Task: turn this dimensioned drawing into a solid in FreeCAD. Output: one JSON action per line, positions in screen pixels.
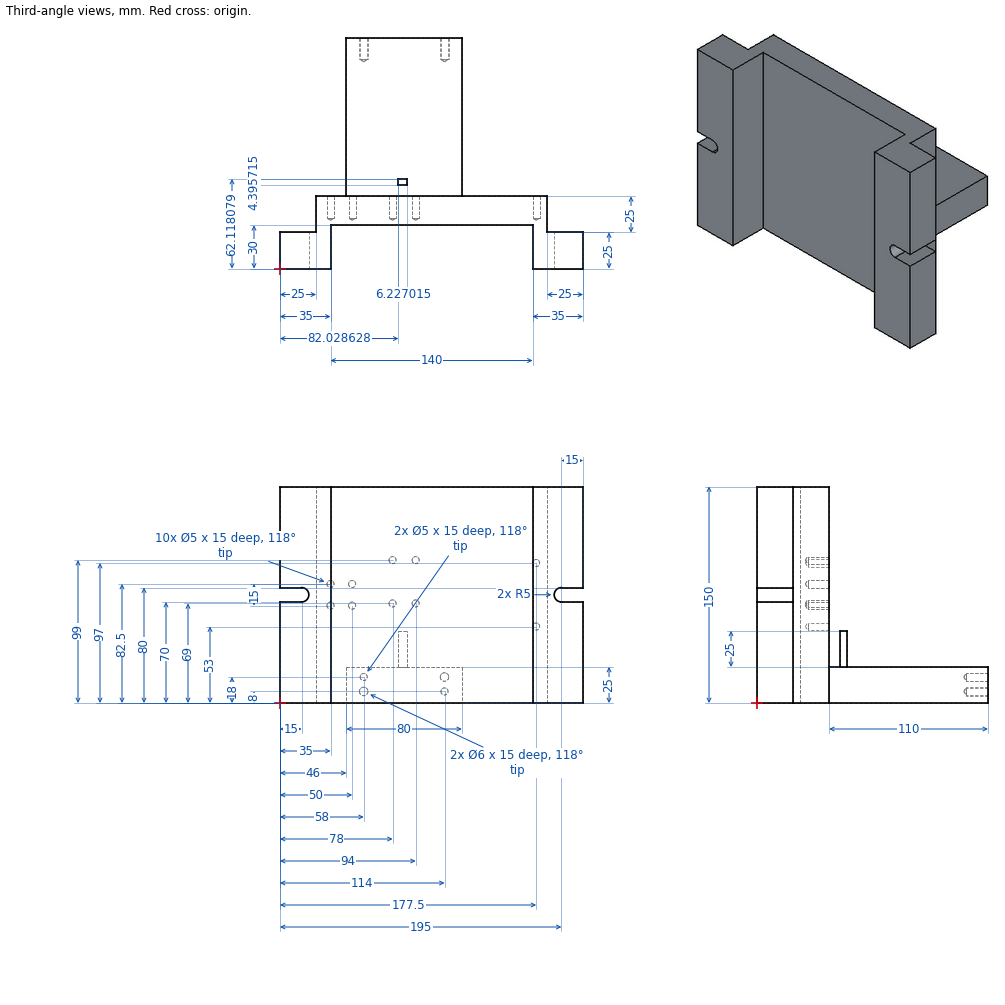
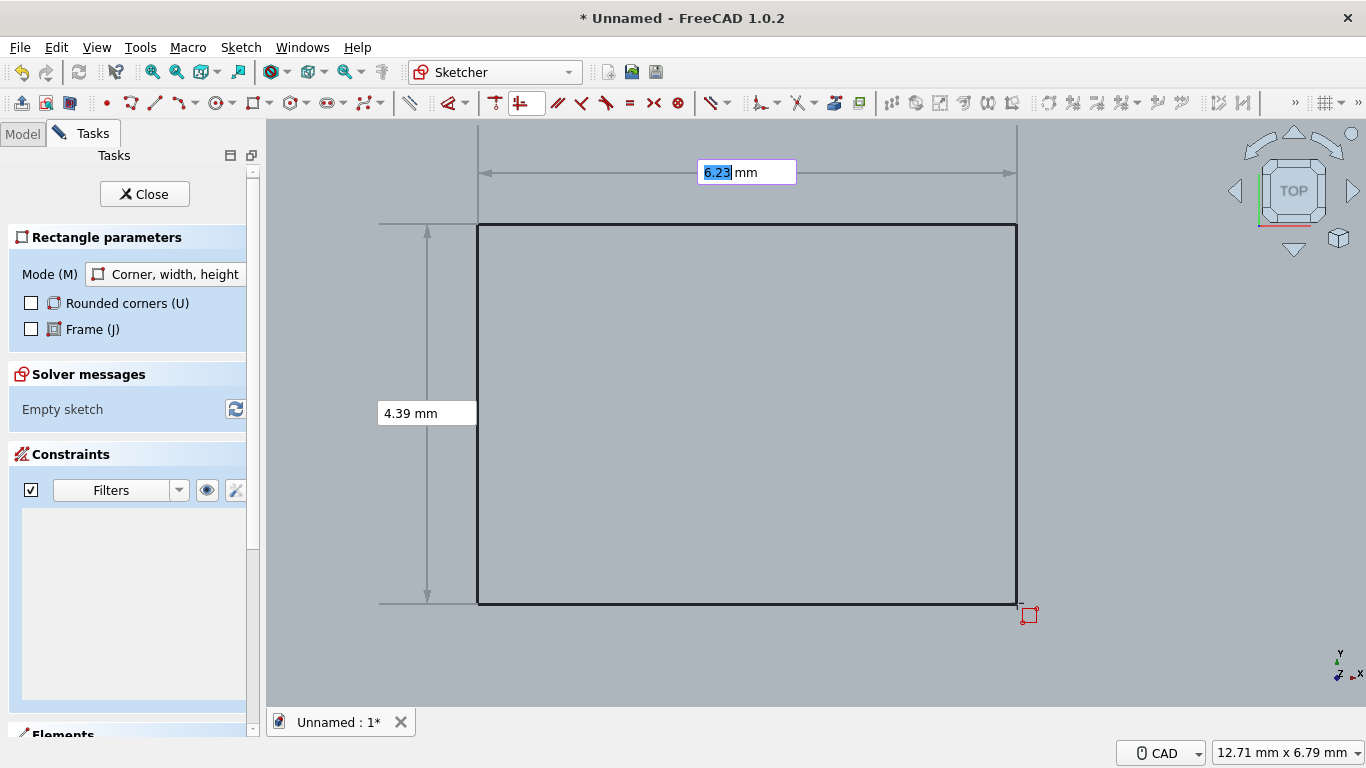
{"action": "type", "text": "6.227015"}
{"action": "key", "text": "Tab"}
{"action": "type", "text": "4.395715"}
{"action": "key", "text": "Return"}
{"action": "key", "text": "Escape"}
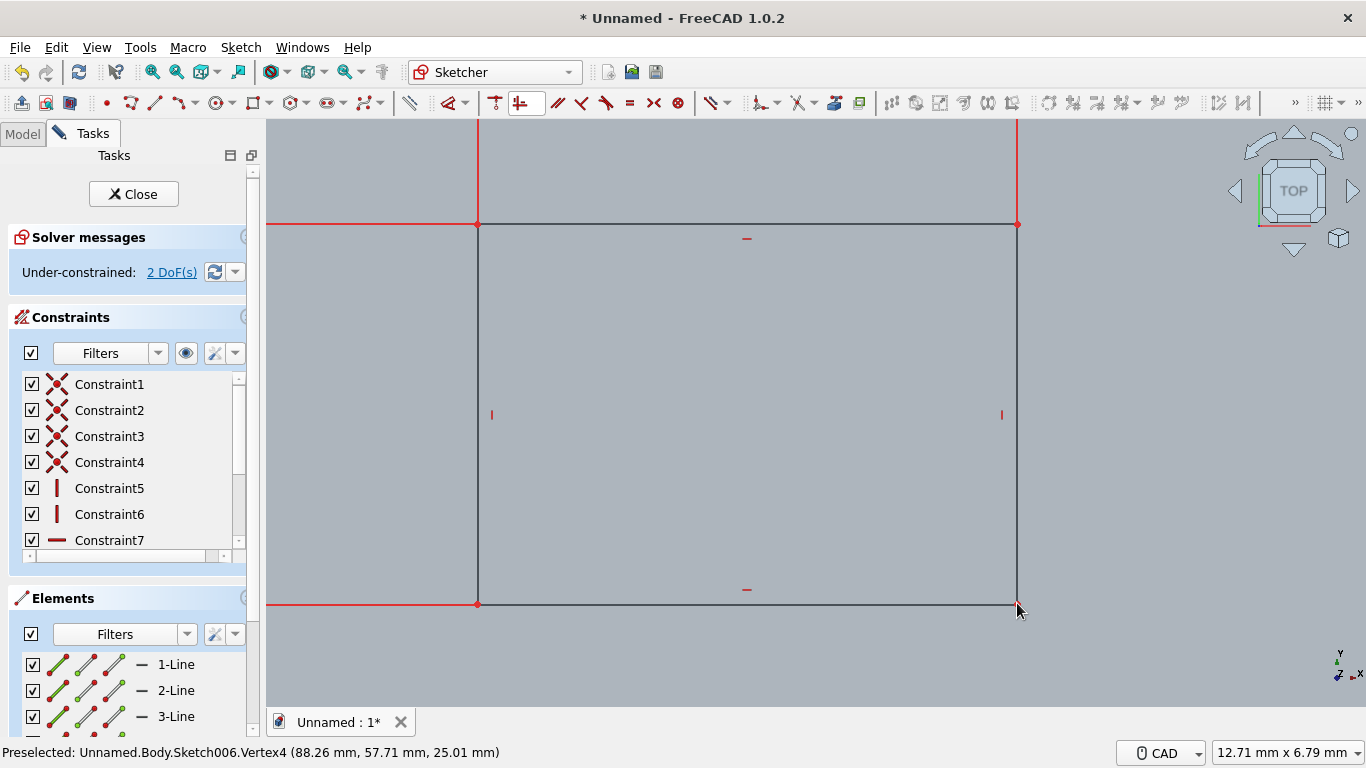
{"action": "key", "text": "d"}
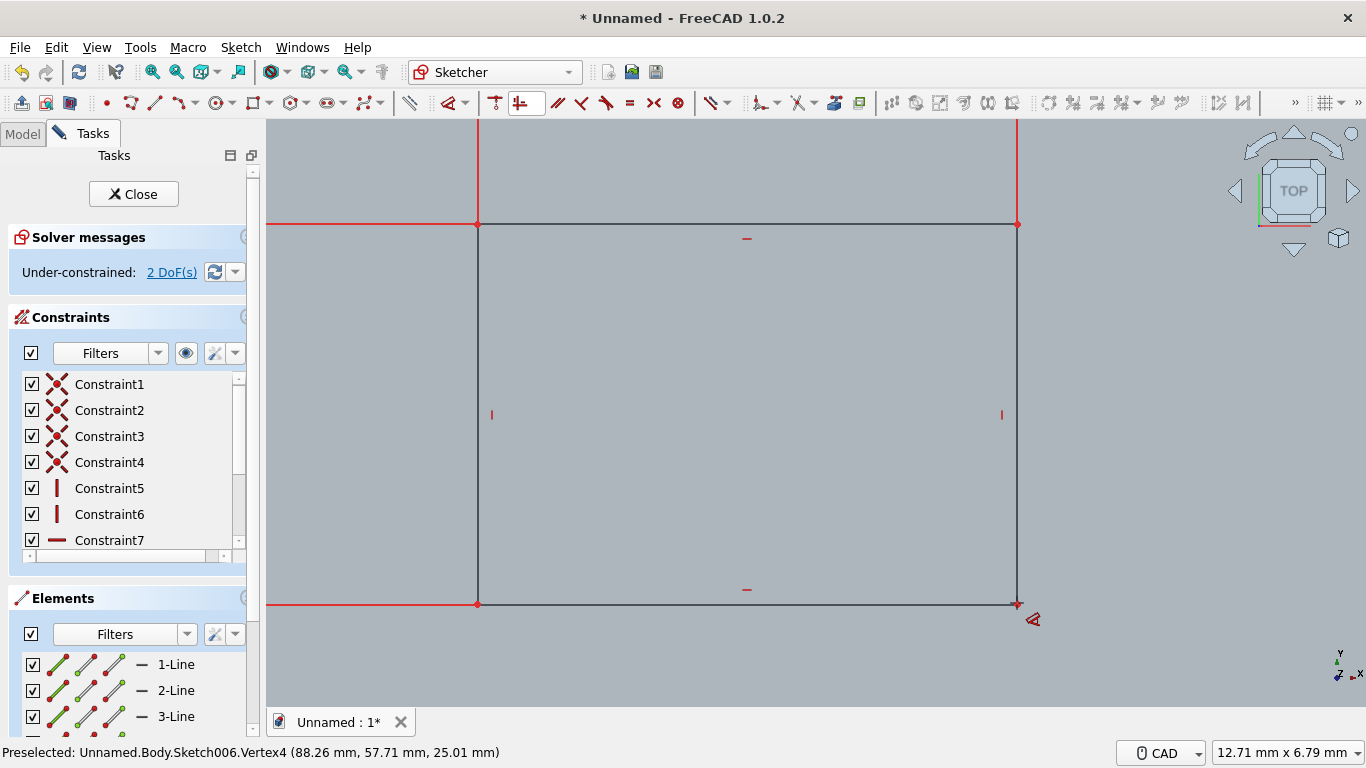
{"action": "left_click", "coordinate": [478, 224]}
{"action": "left_click", "coordinate": [386, 190]}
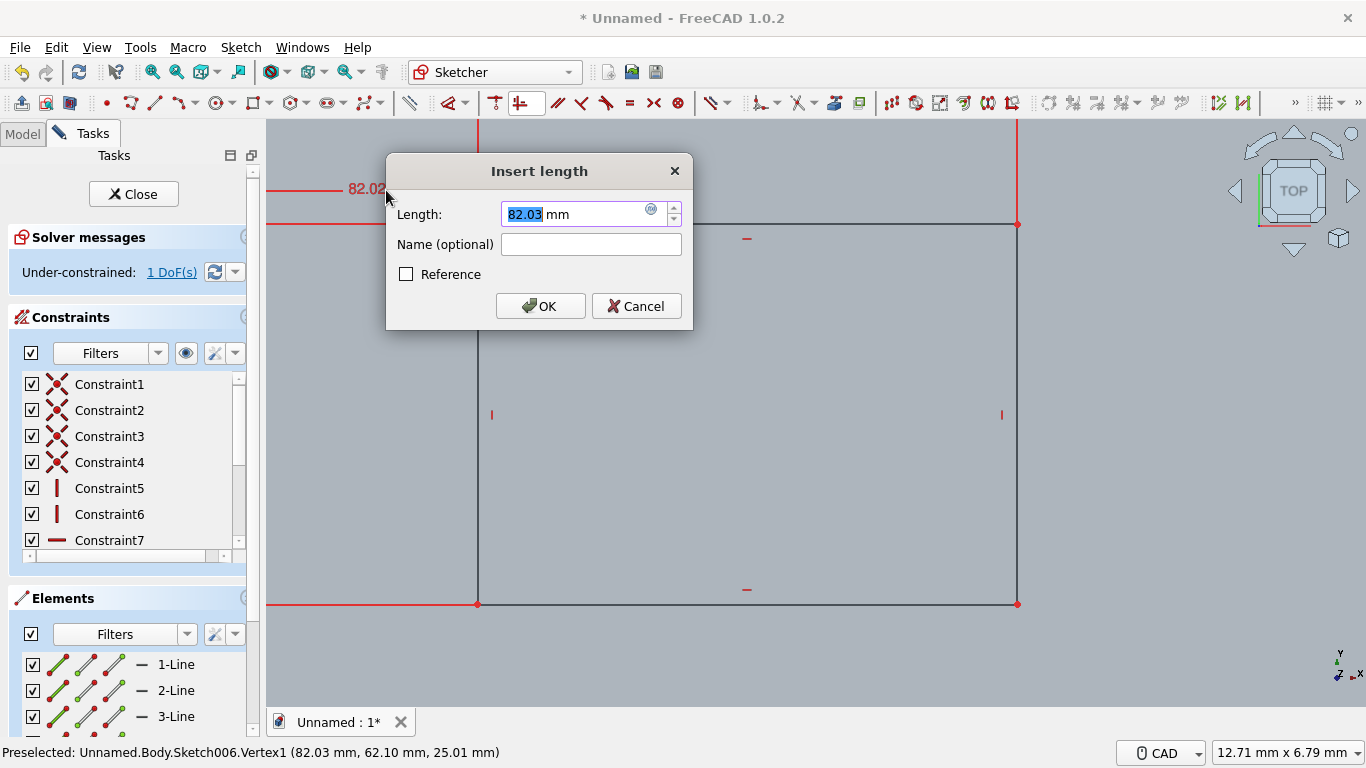
{"action": "type", "text": "82.028628"}
{"action": "key", "text": "Return"}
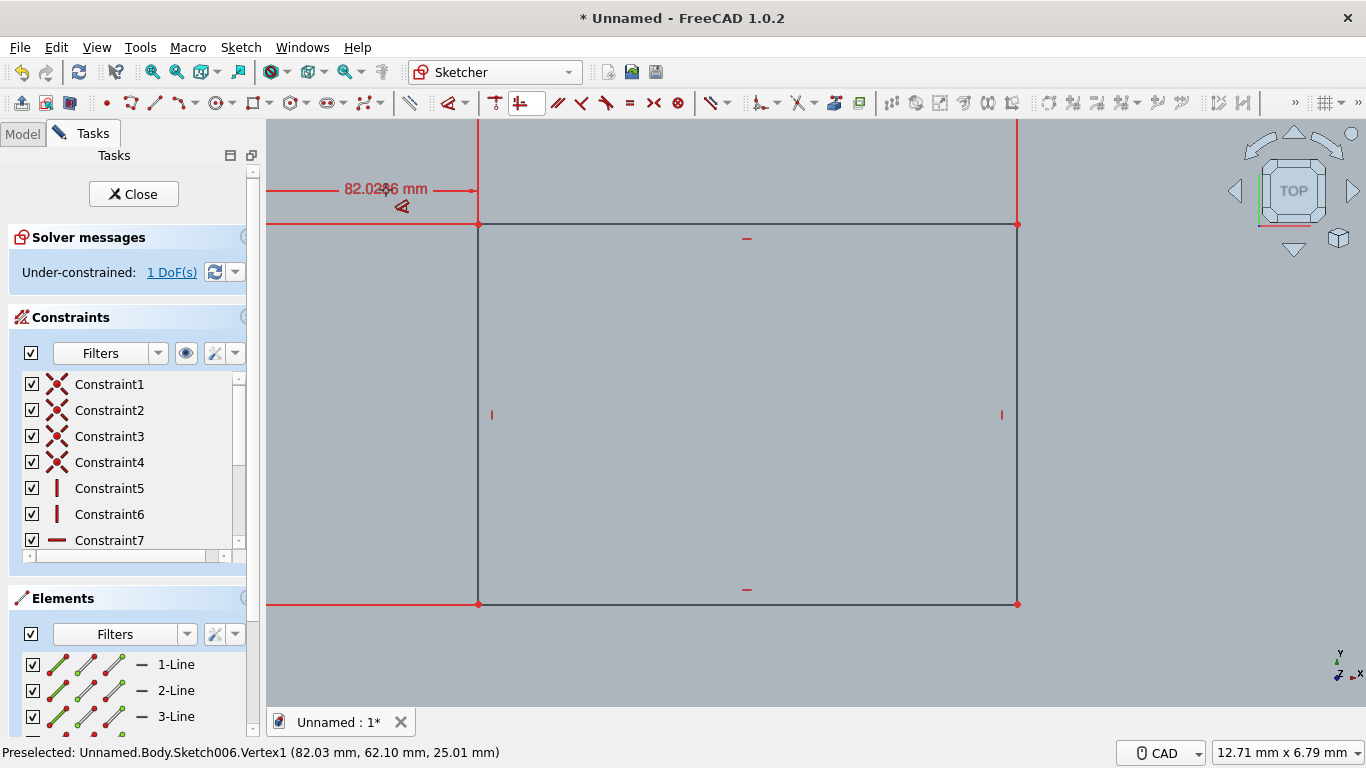
{"action": "left_click", "coordinate": [478, 224]}
{"action": "left_click", "coordinate": [512, 452]}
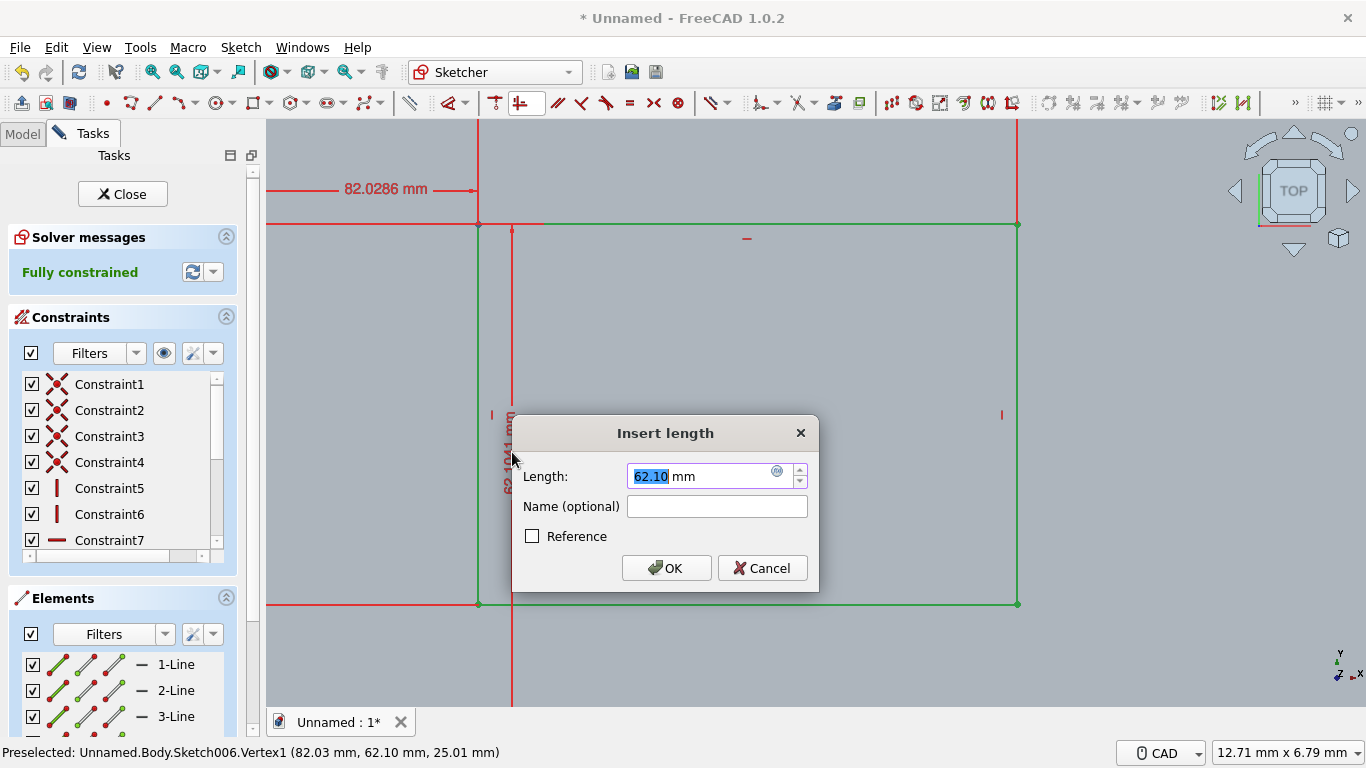
{"action": "type", "text": "62.118079"}
{"action": "key", "text": "Return"}
{"action": "key", "text": "Escape"}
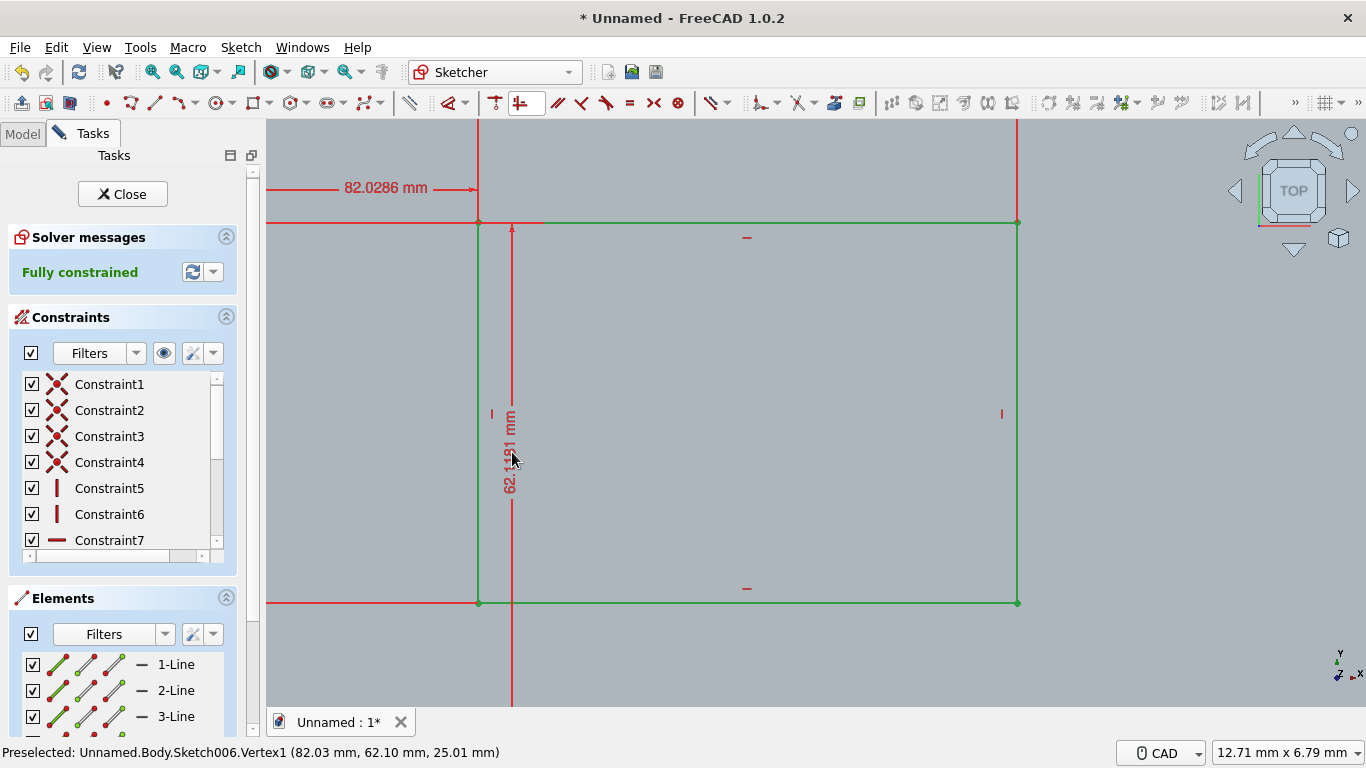
{"action": "left_click", "coordinate": [123, 194]}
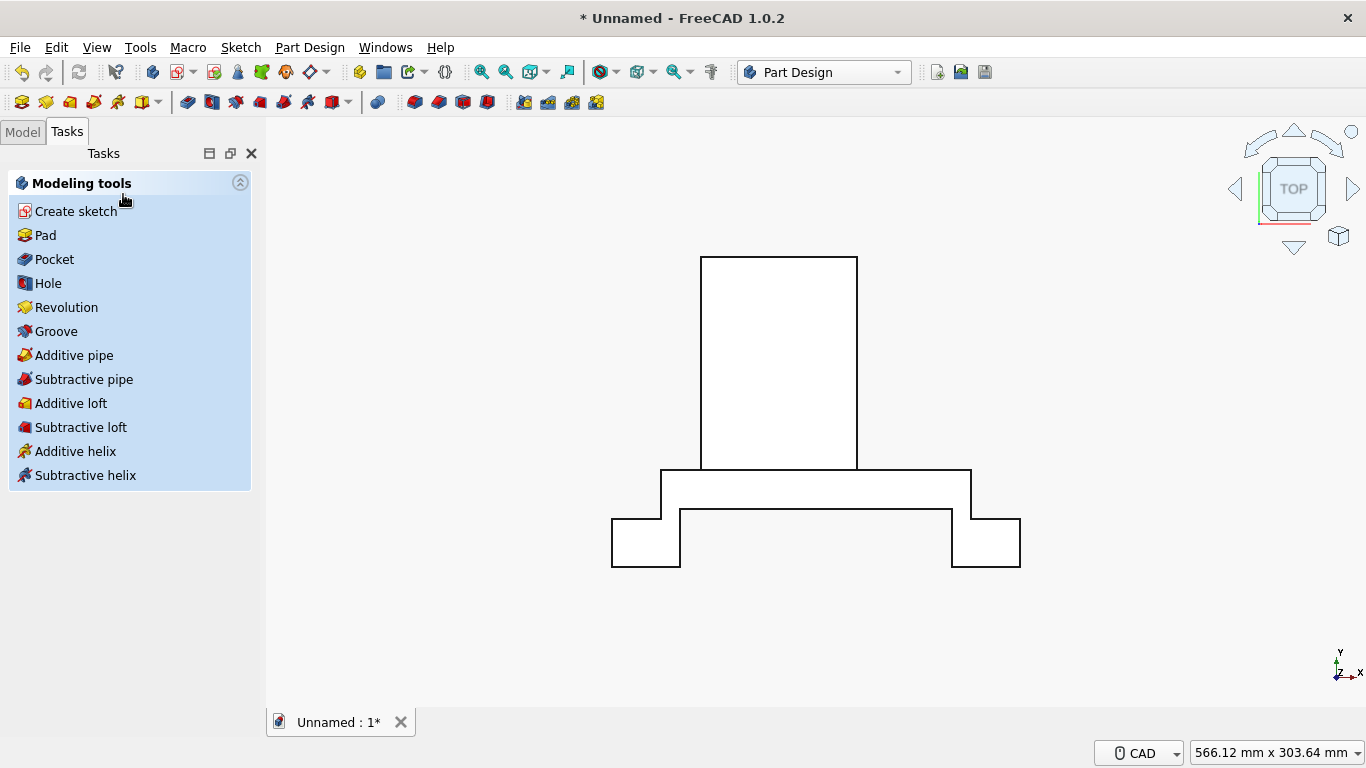
{"action": "left_click", "coordinate": [22, 102]}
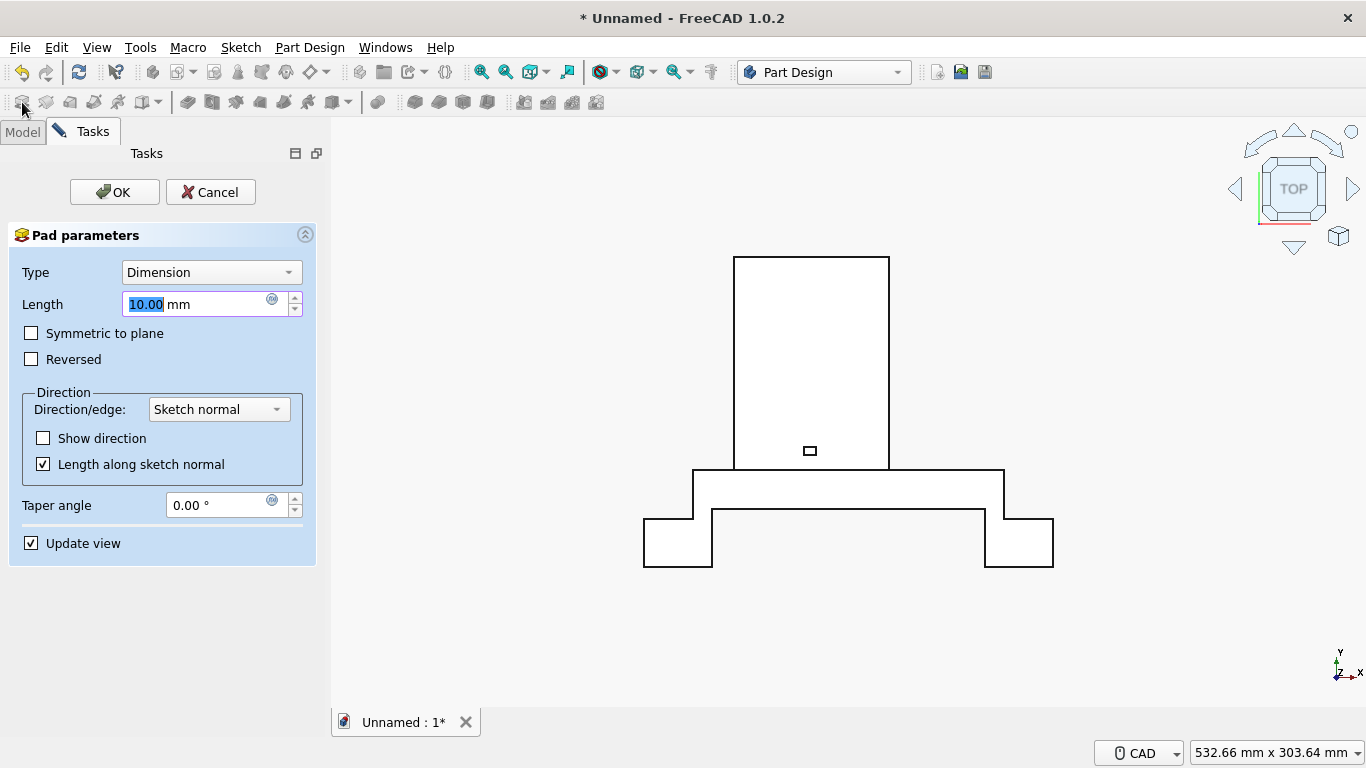
{"action": "type", "text": "25"}
{"action": "key", "text": "Tab"}